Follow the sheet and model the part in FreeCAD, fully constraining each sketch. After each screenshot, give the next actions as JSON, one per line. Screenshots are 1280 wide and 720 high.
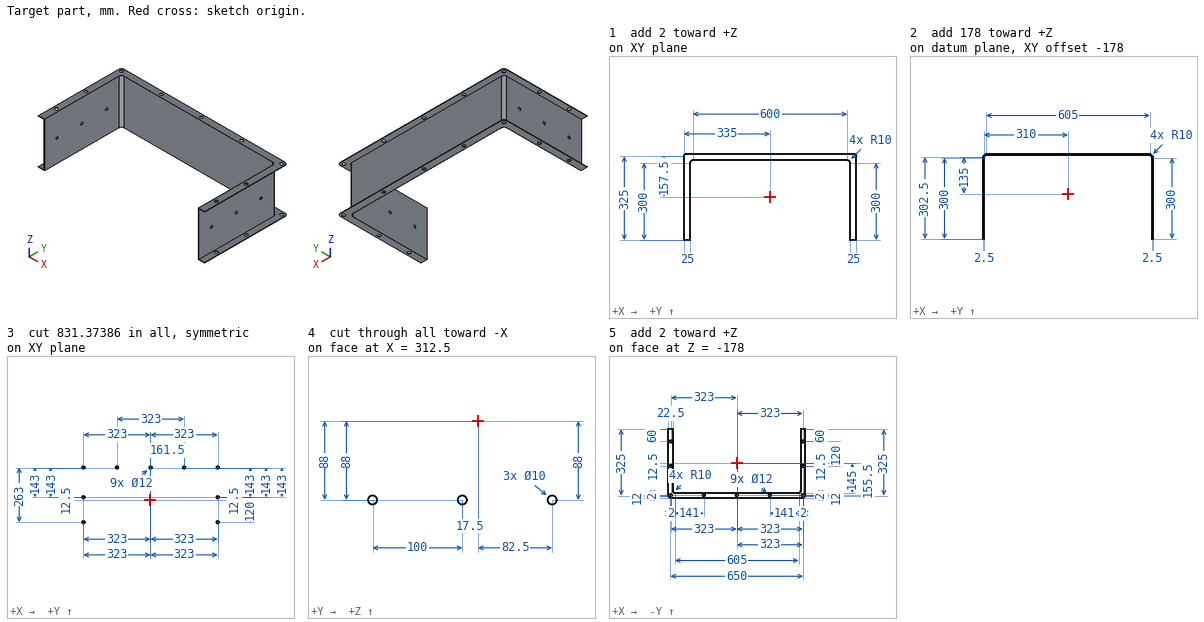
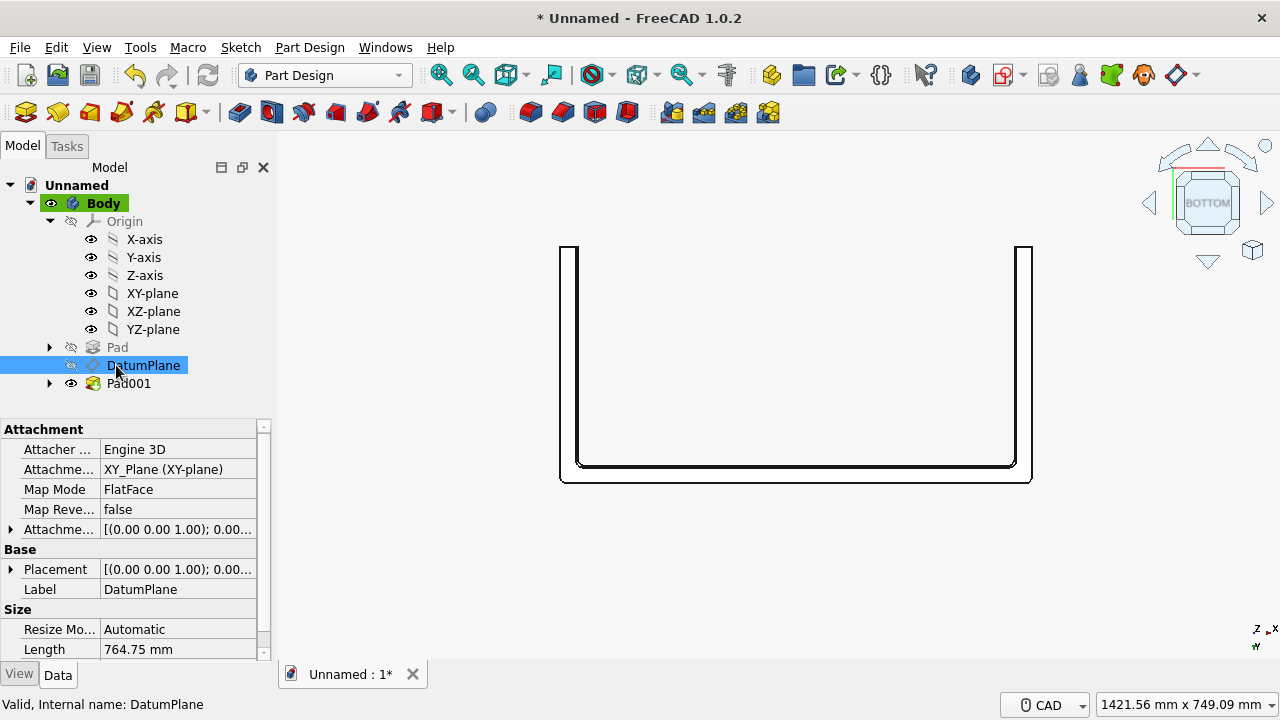
{"action": "key", "text": "1"}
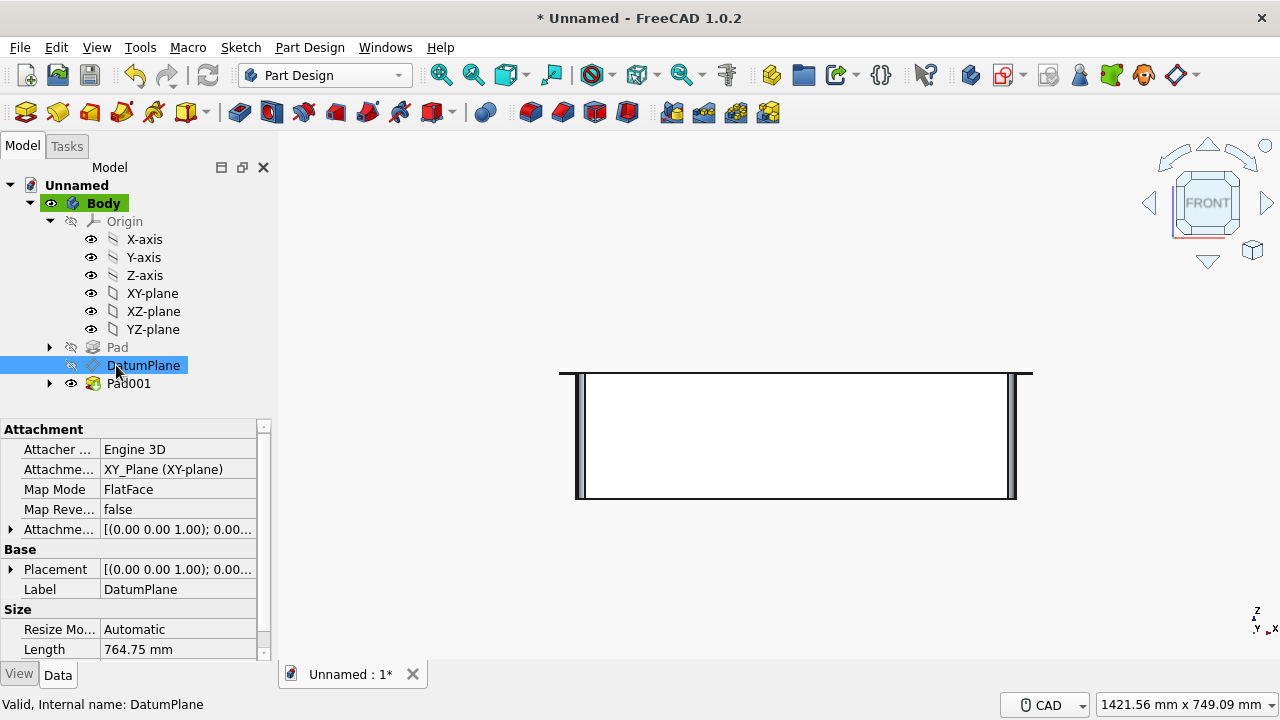
{"action": "key", "text": "3"}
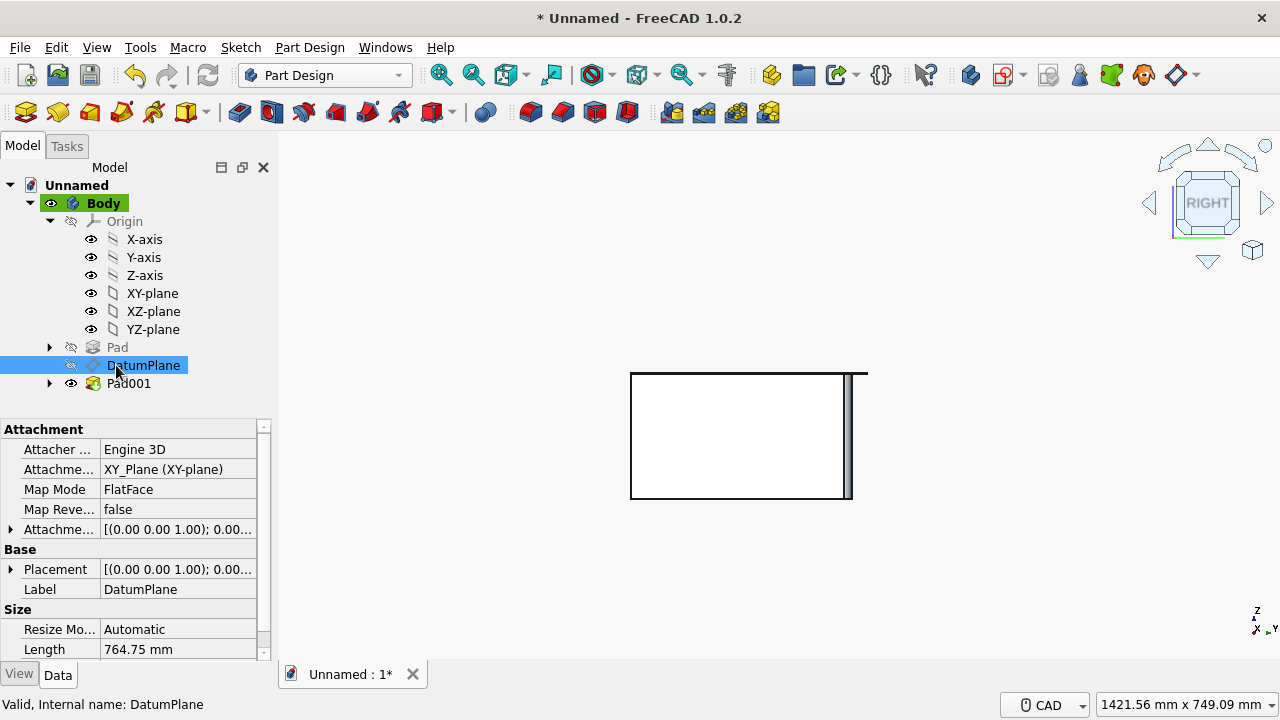
{"action": "left_click", "coordinate": [442, 76]}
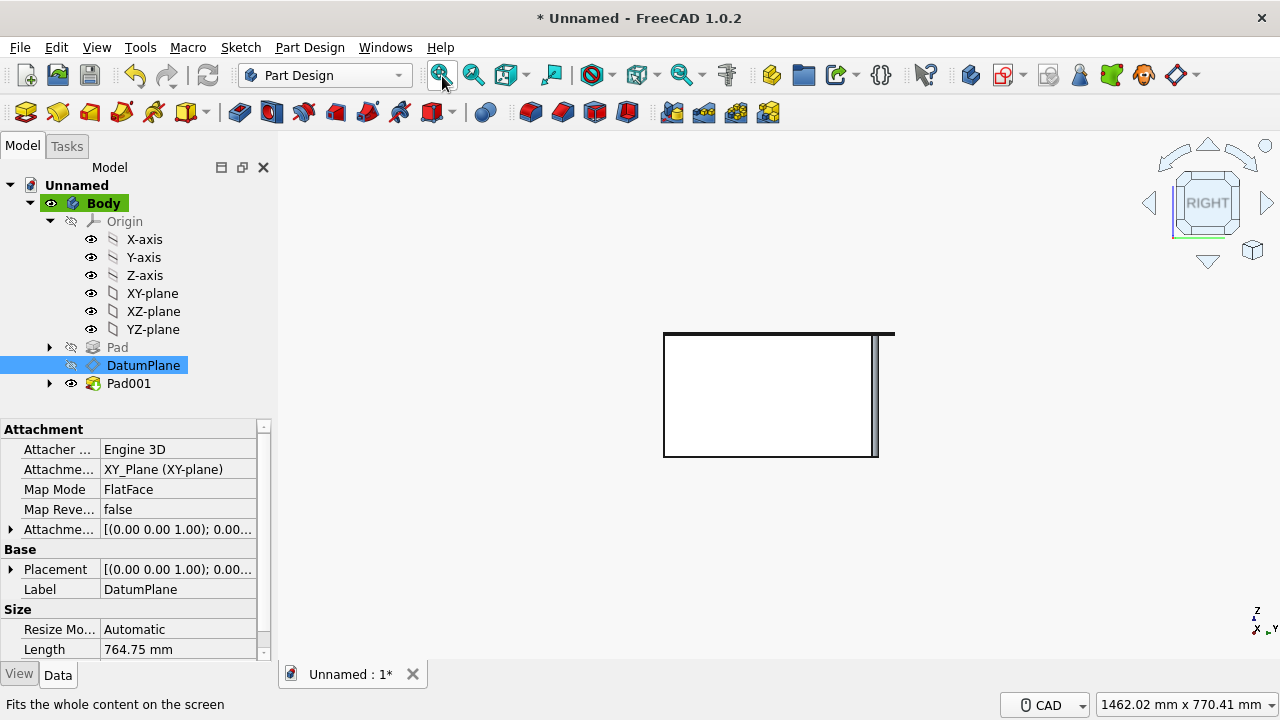
{"action": "left_click", "coordinate": [318, 619]}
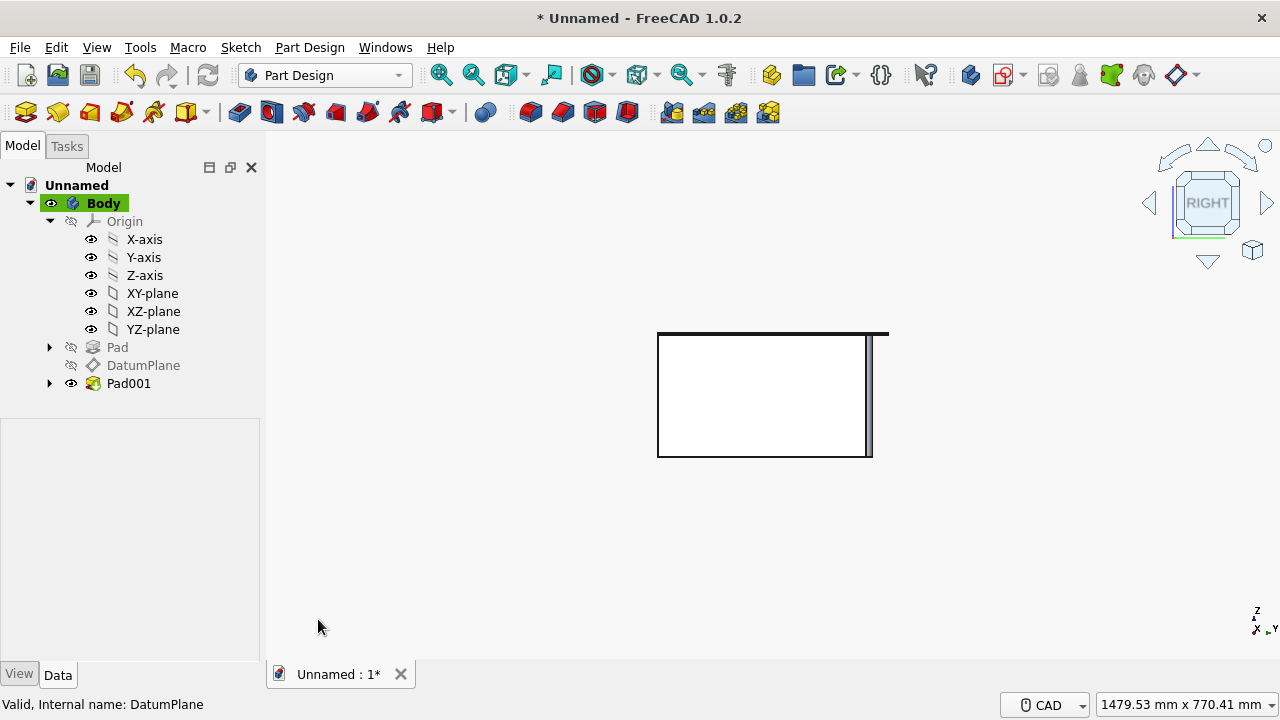
{"action": "left_click", "coordinate": [1004, 76]}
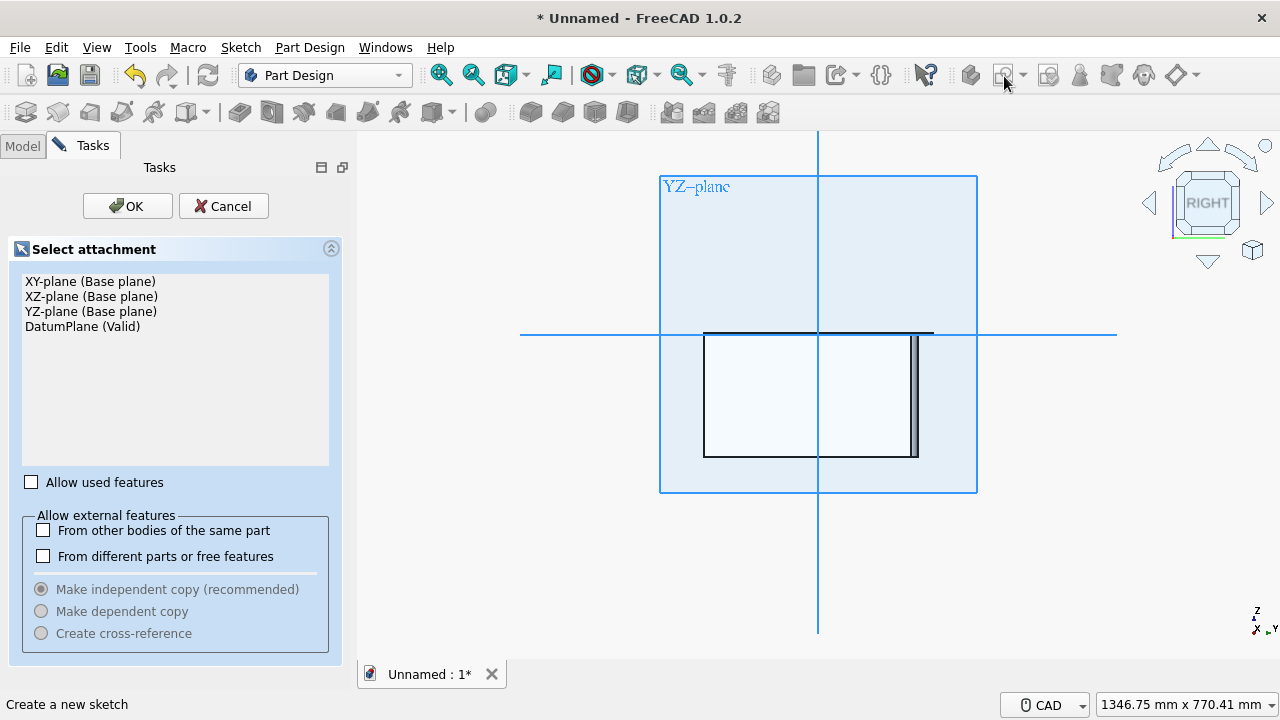
{"action": "left_click", "coordinate": [82, 282]}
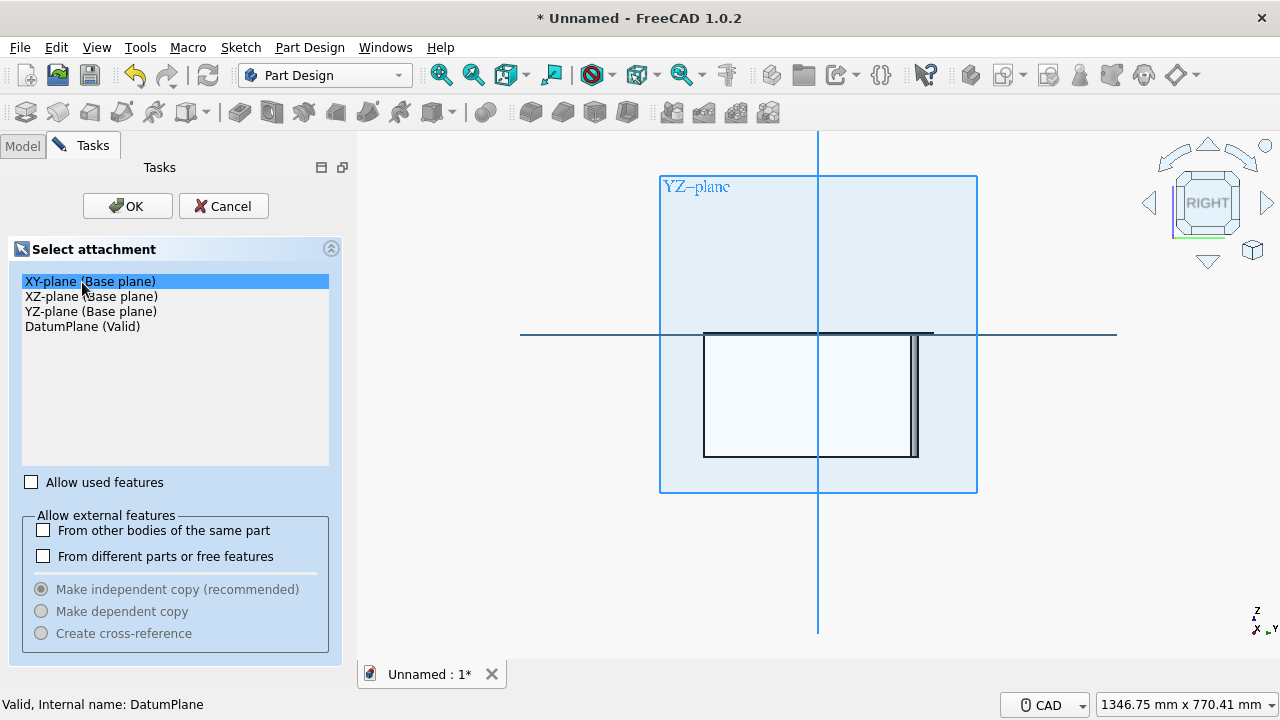
{"action": "left_click", "coordinate": [128, 206]}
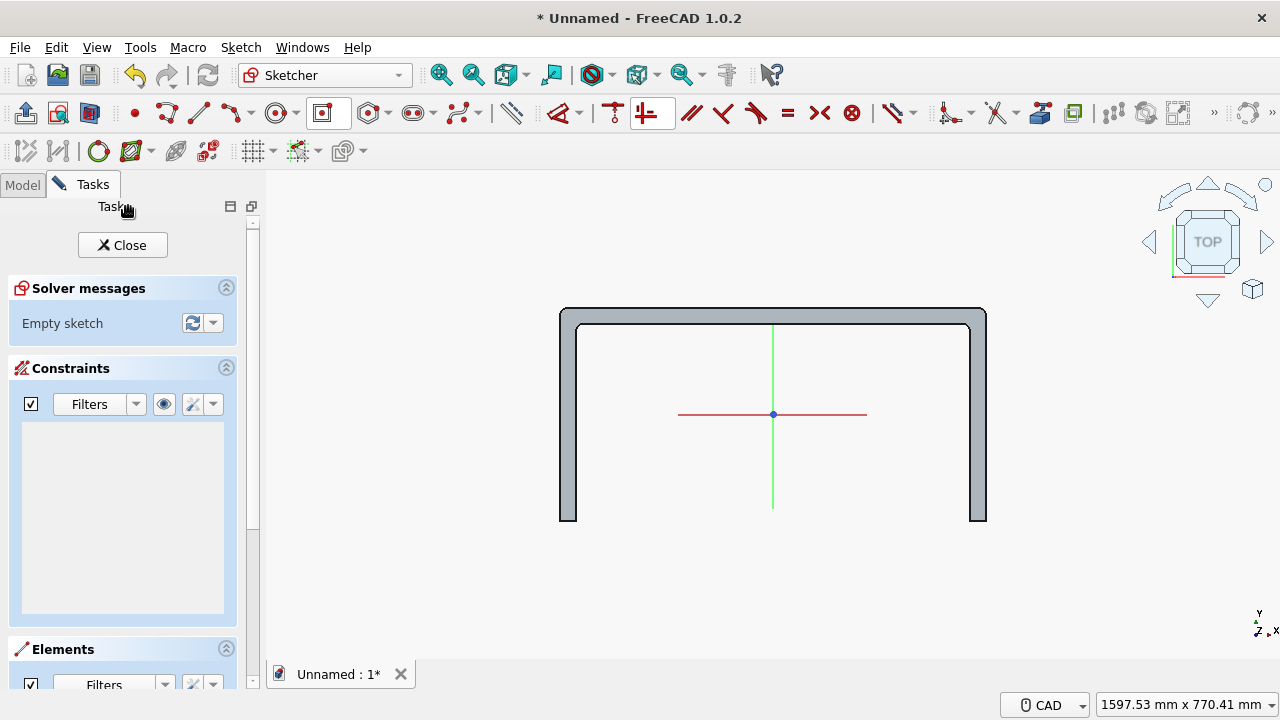
{"action": "left_click", "coordinate": [90, 114]}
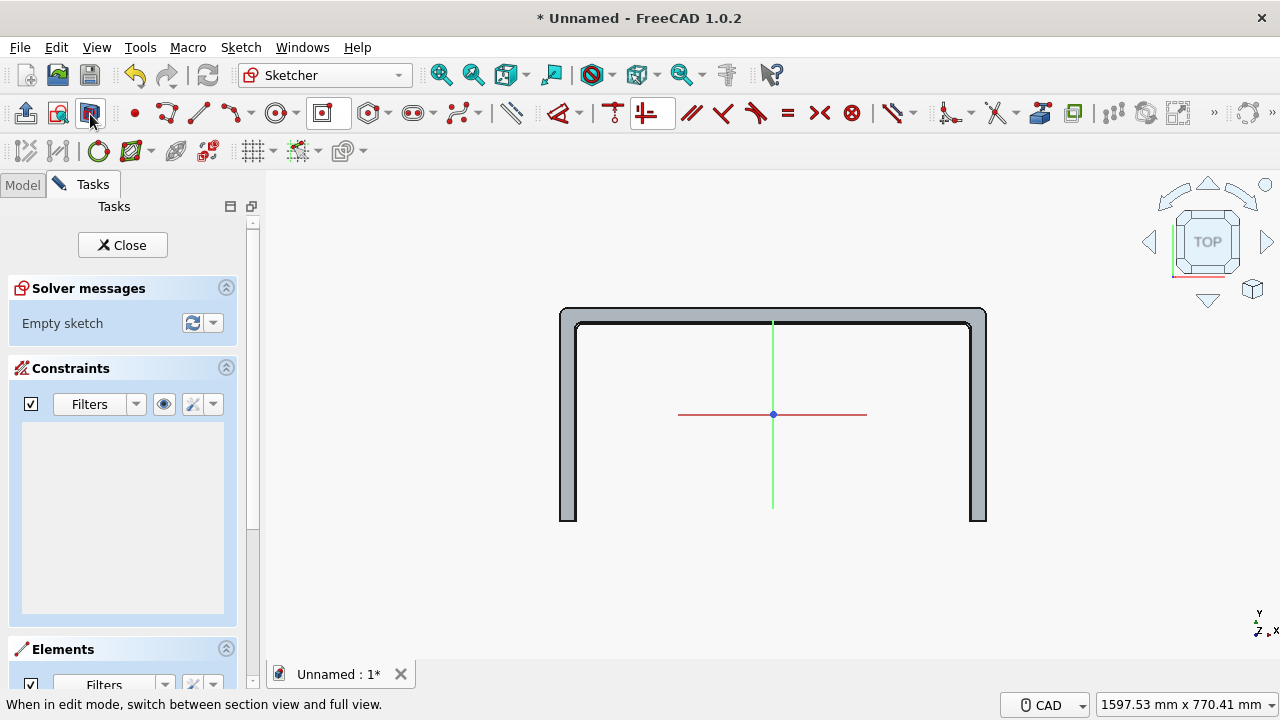
{"action": "scroll", "coordinate": [912, 368], "scroll_direction": "up", "scroll_amount": 2}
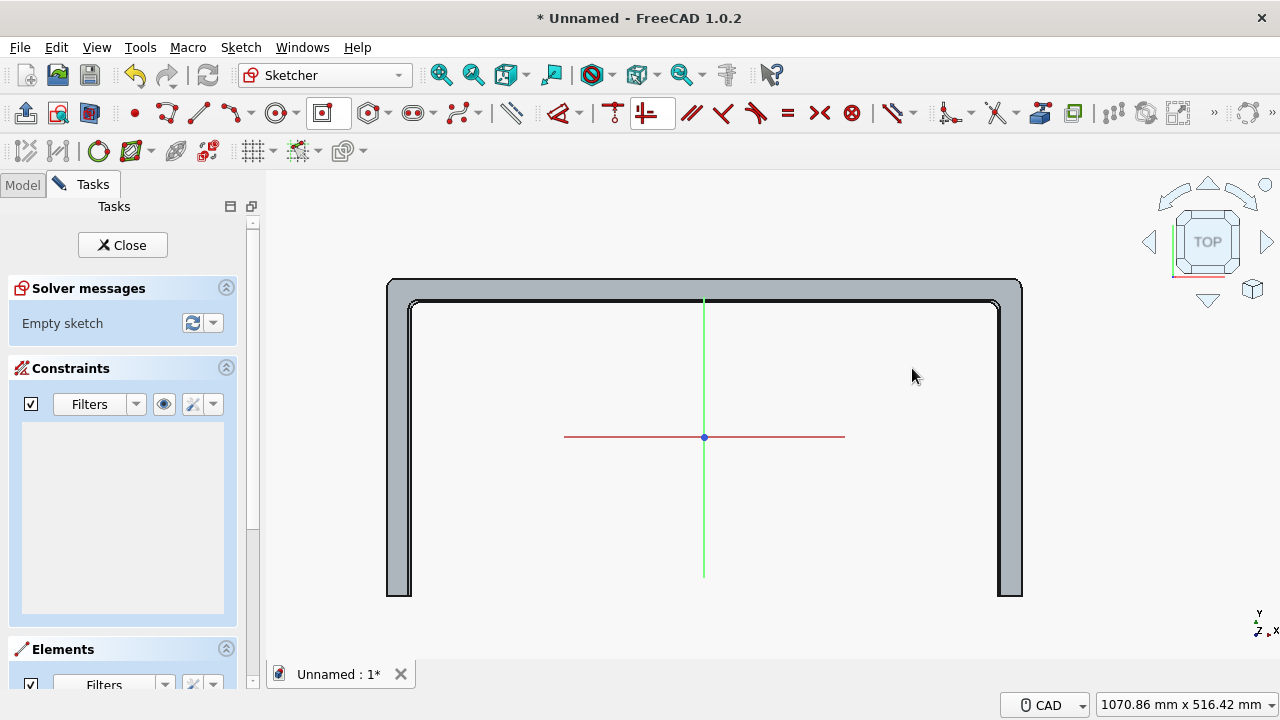
{"action": "left_click", "coordinate": [276, 114]}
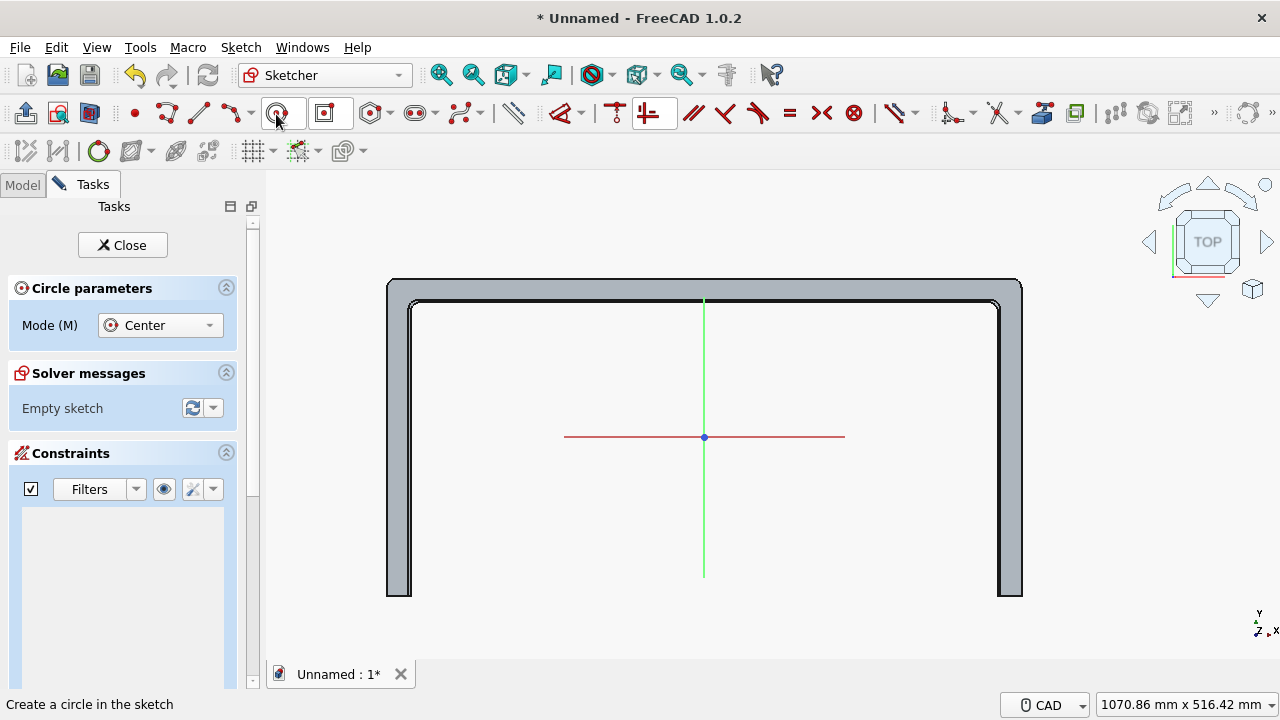
{"action": "scroll", "coordinate": [704, 290], "scroll_direction": "up", "scroll_amount": 7}